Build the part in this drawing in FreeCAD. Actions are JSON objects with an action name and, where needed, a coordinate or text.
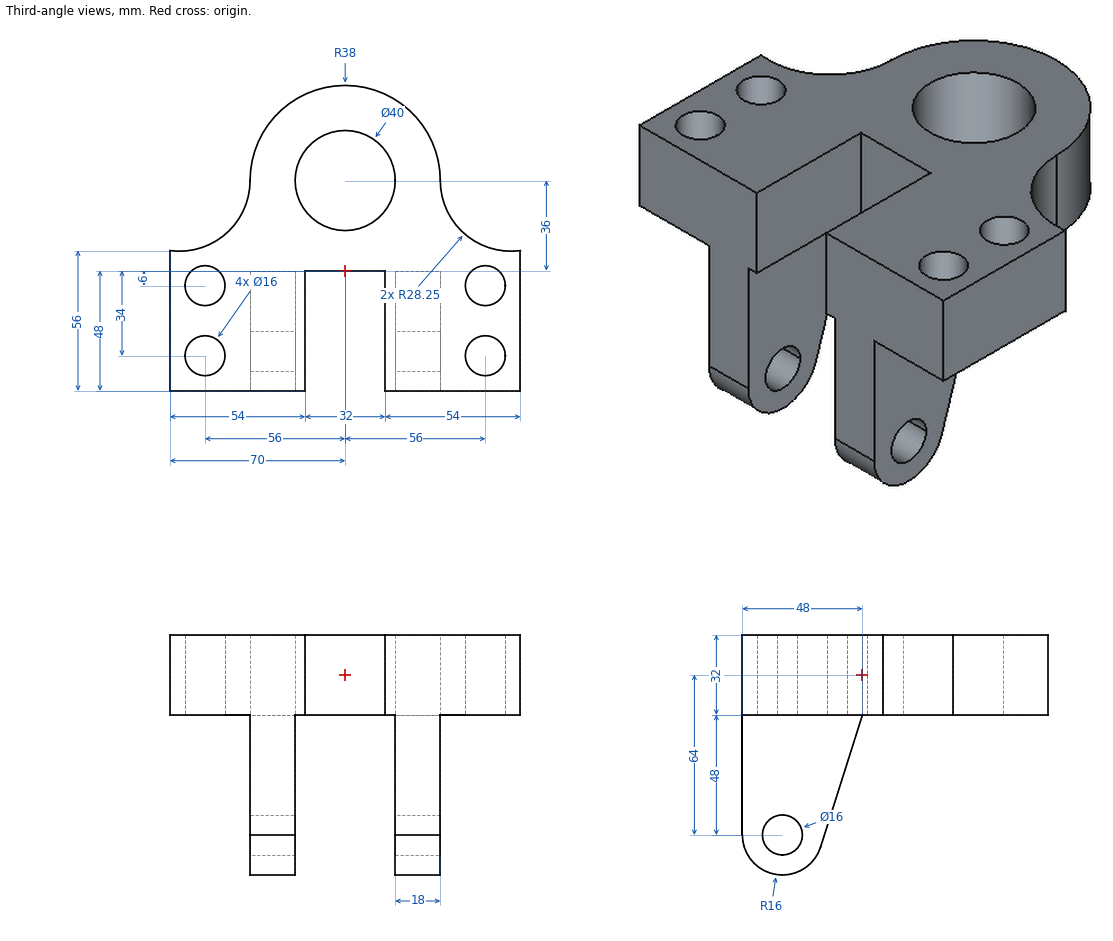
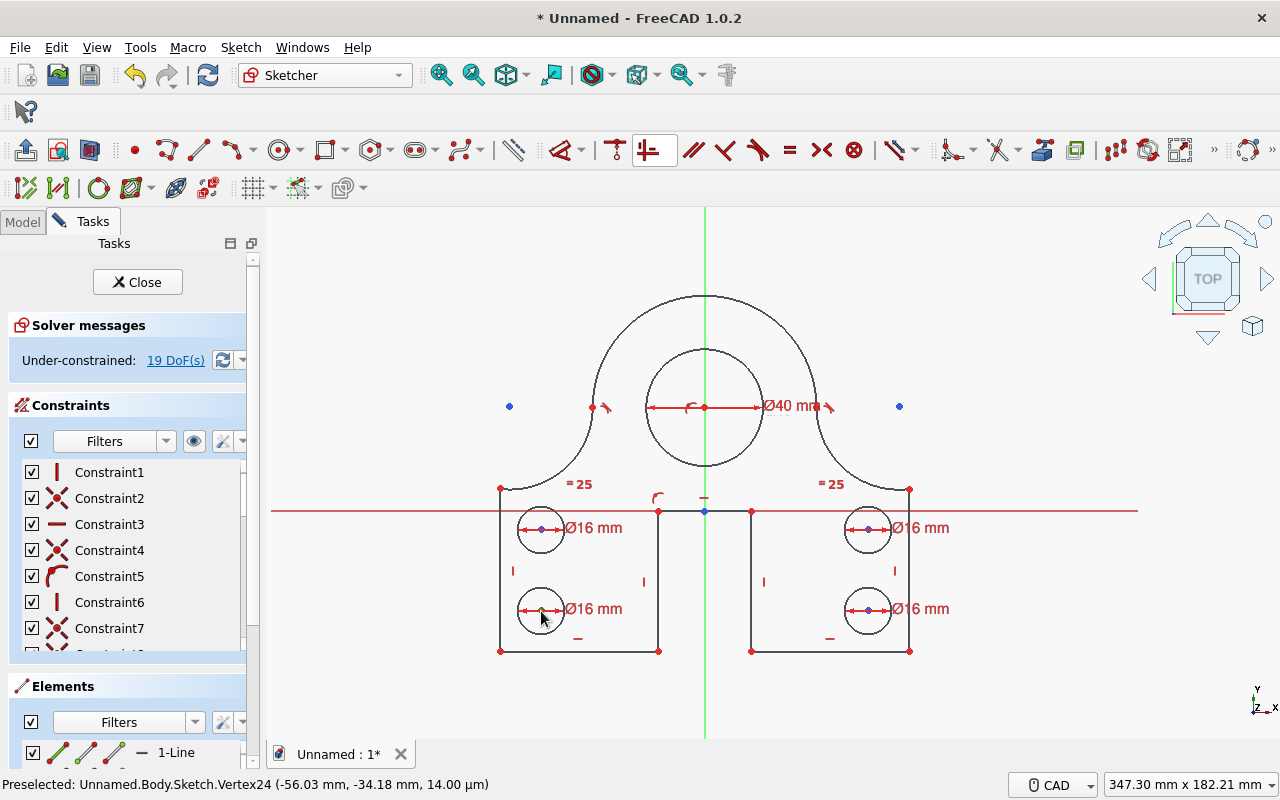
{"action": "left_click", "coordinate": [541, 530]}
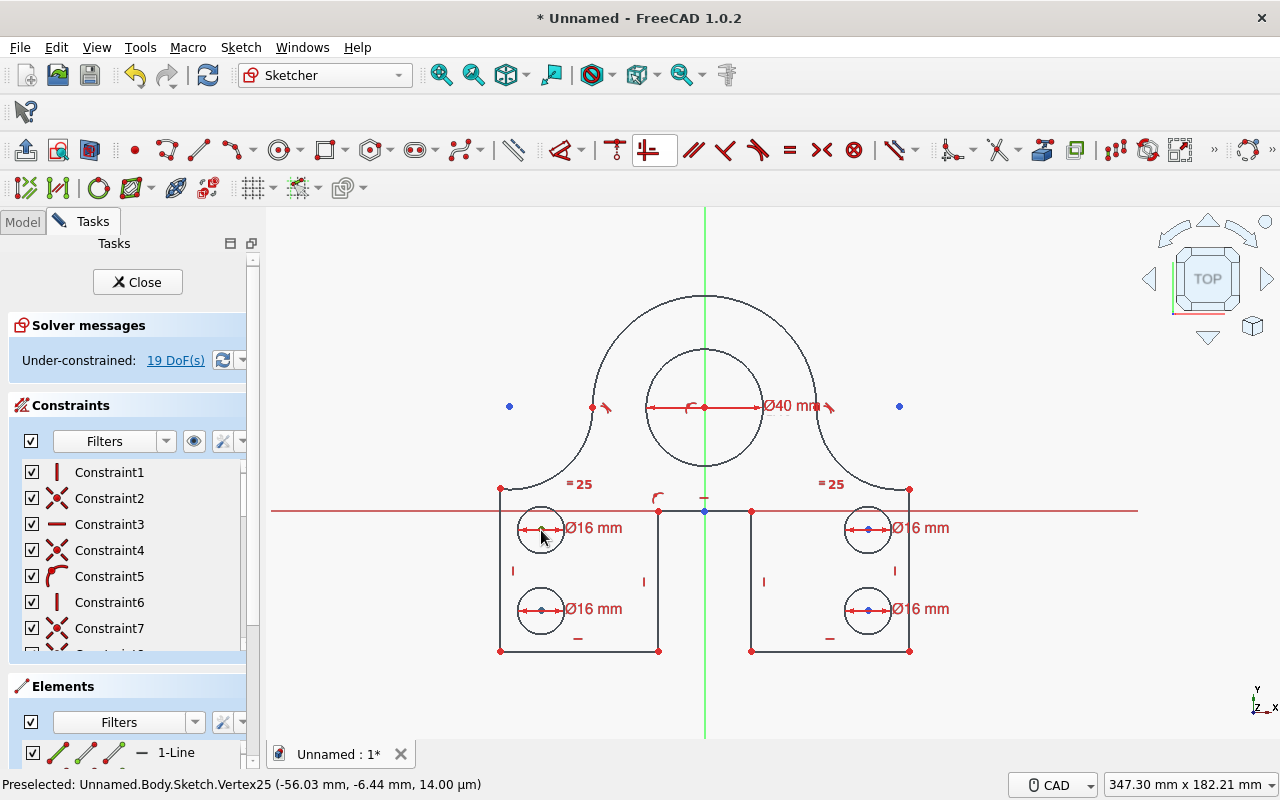
{"action": "key", "text": "v"}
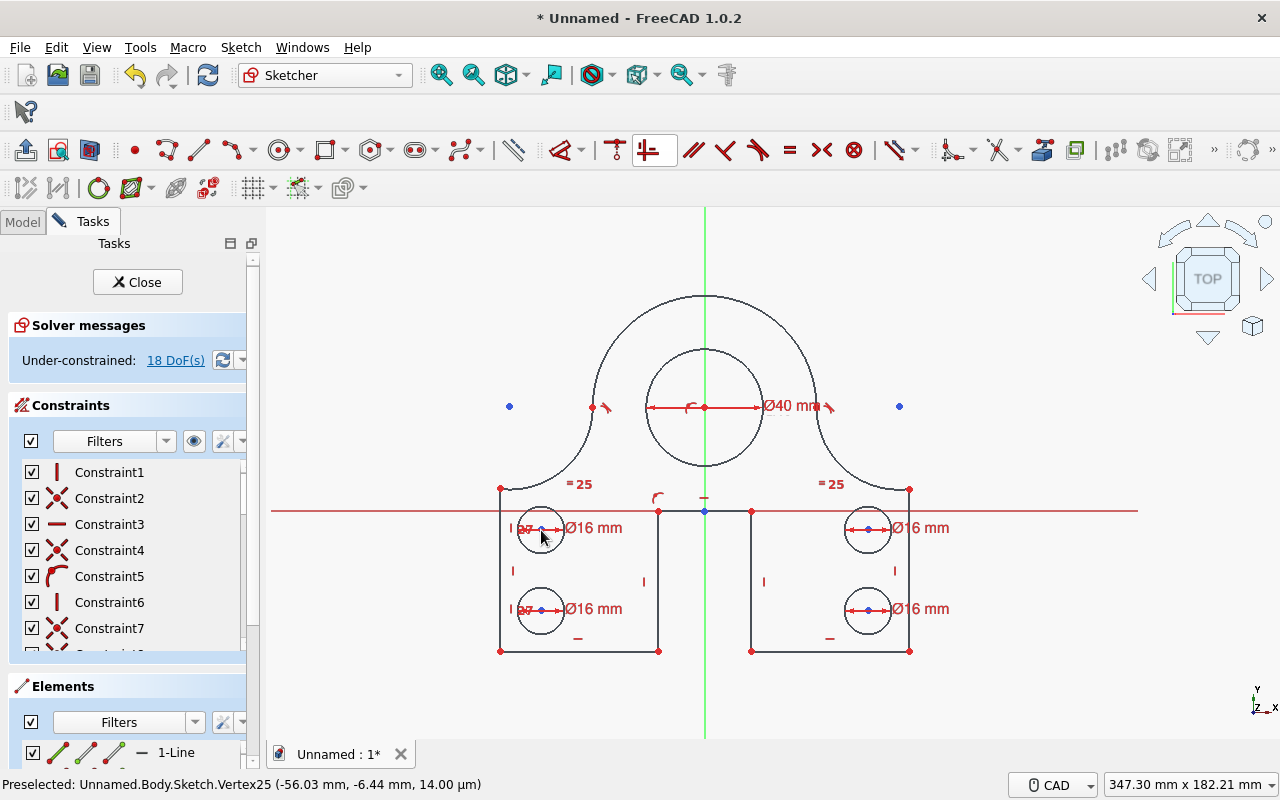
{"action": "left_click", "coordinate": [868, 611]}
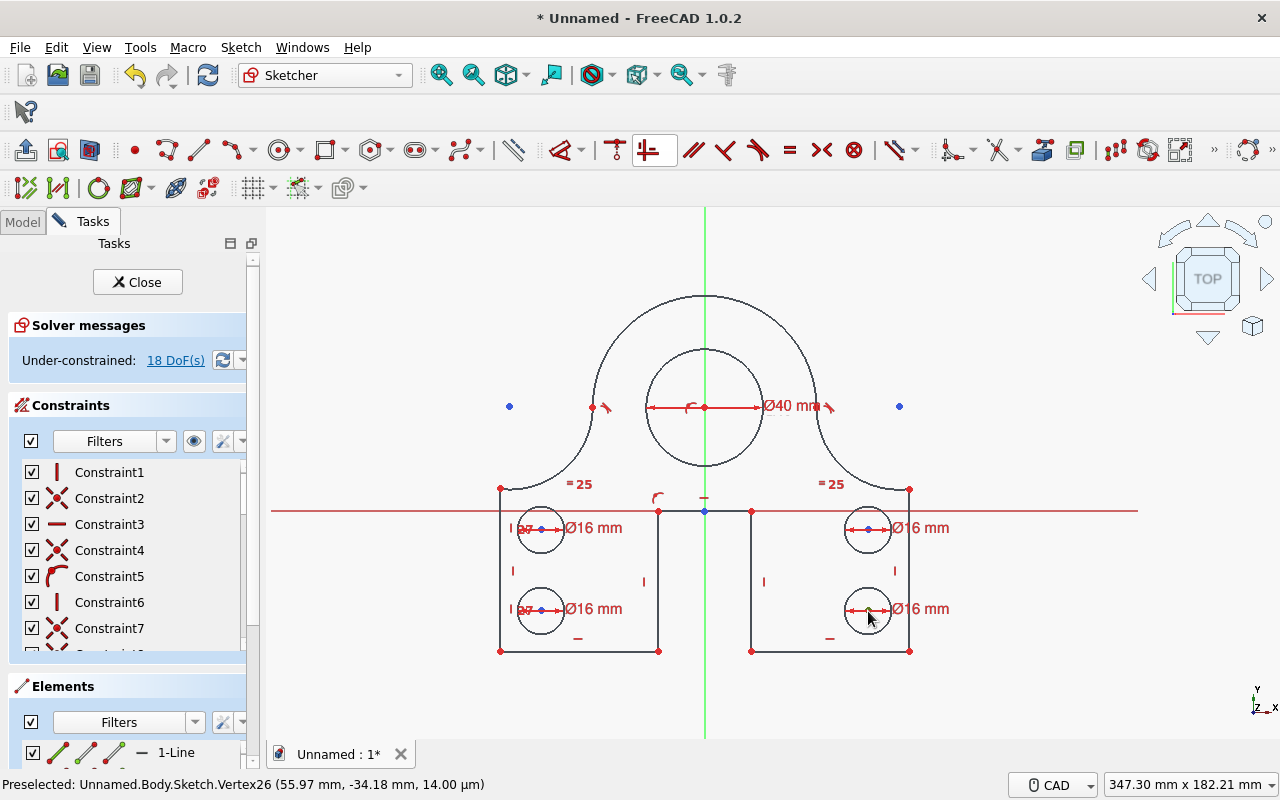
{"action": "left_click", "coordinate": [868, 530]}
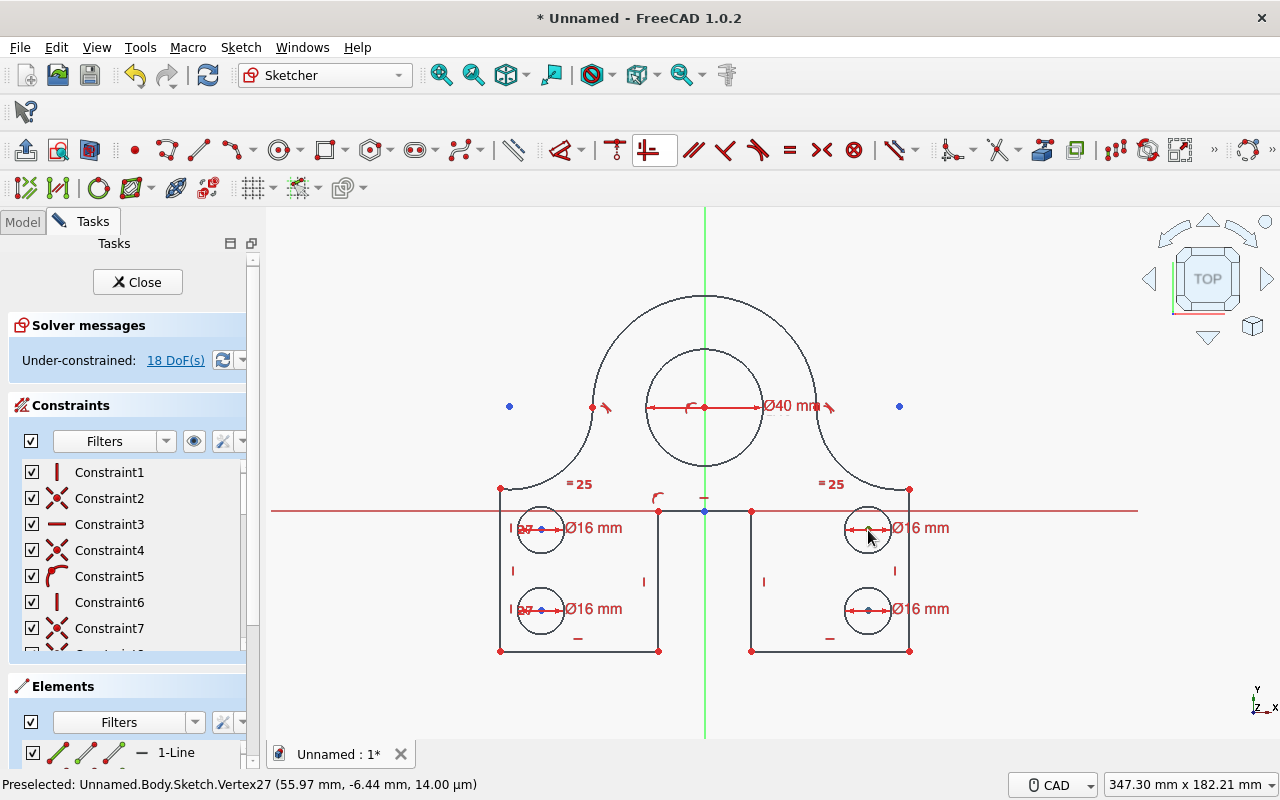
{"action": "left_click", "coordinate": [672, 150]}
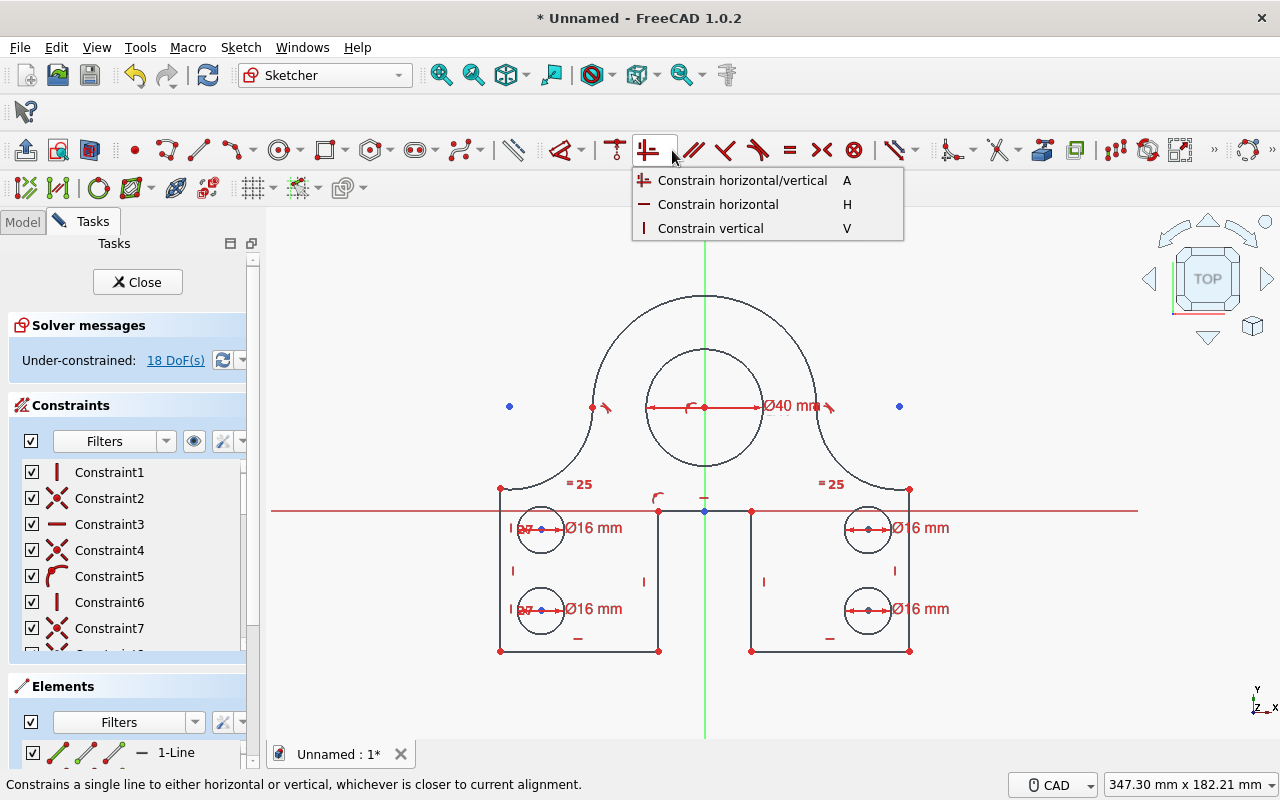
{"action": "left_click", "coordinate": [768, 228]}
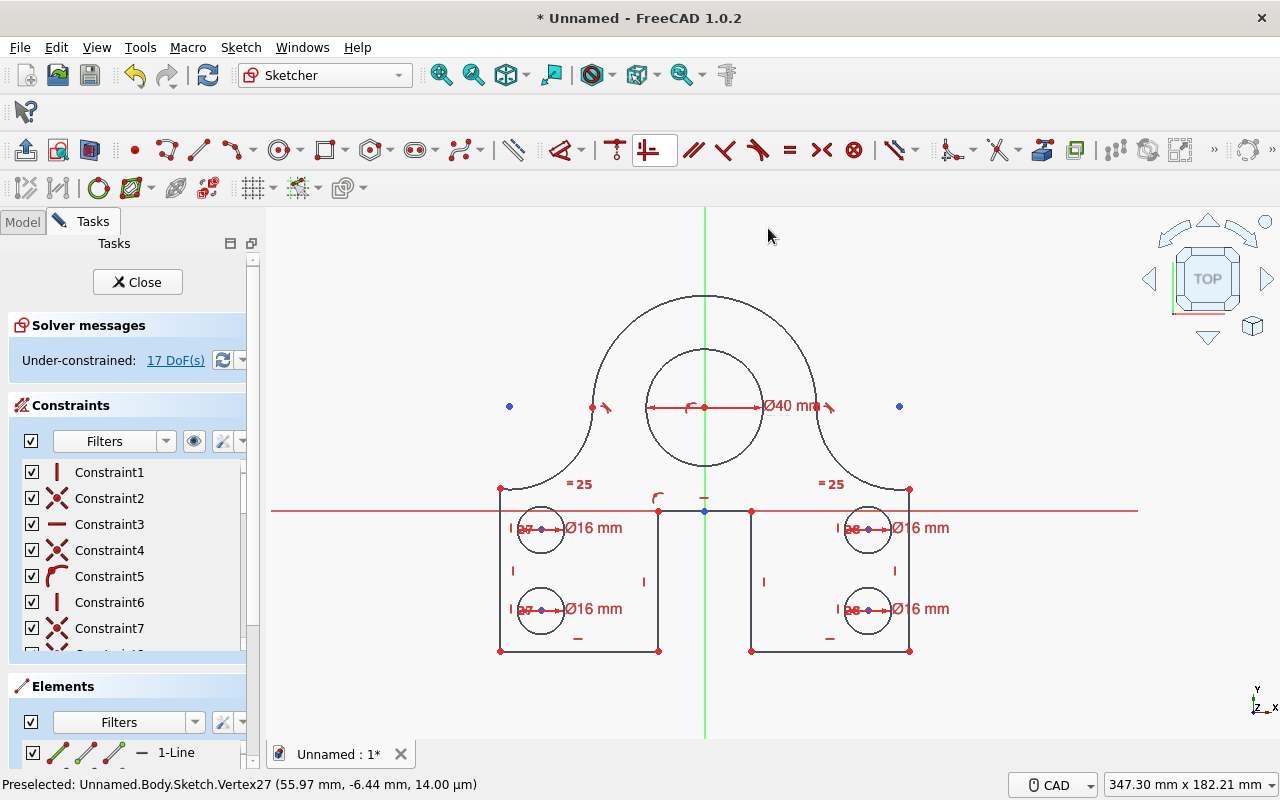
{"action": "left_click", "coordinate": [560, 150]}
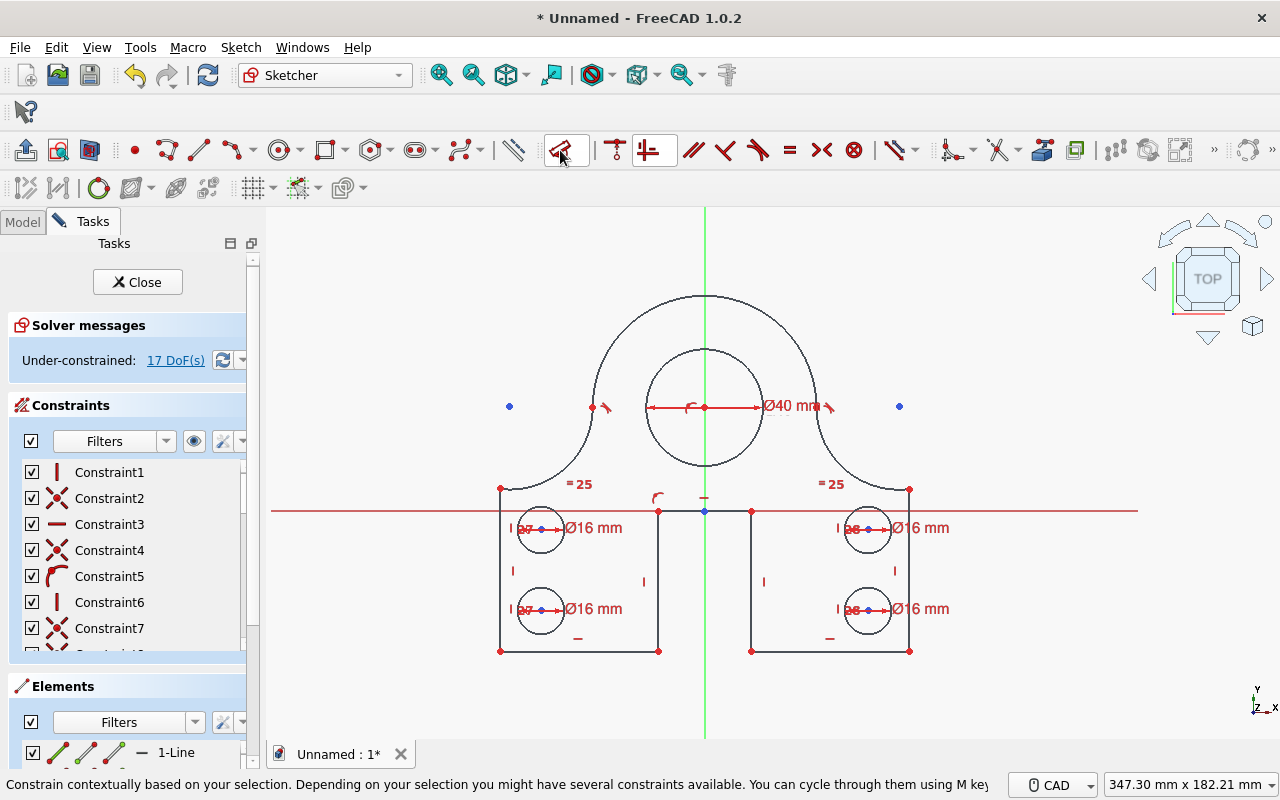
{"action": "left_click", "coordinate": [827, 447]}
{"action": "left_click", "coordinate": [799, 463]}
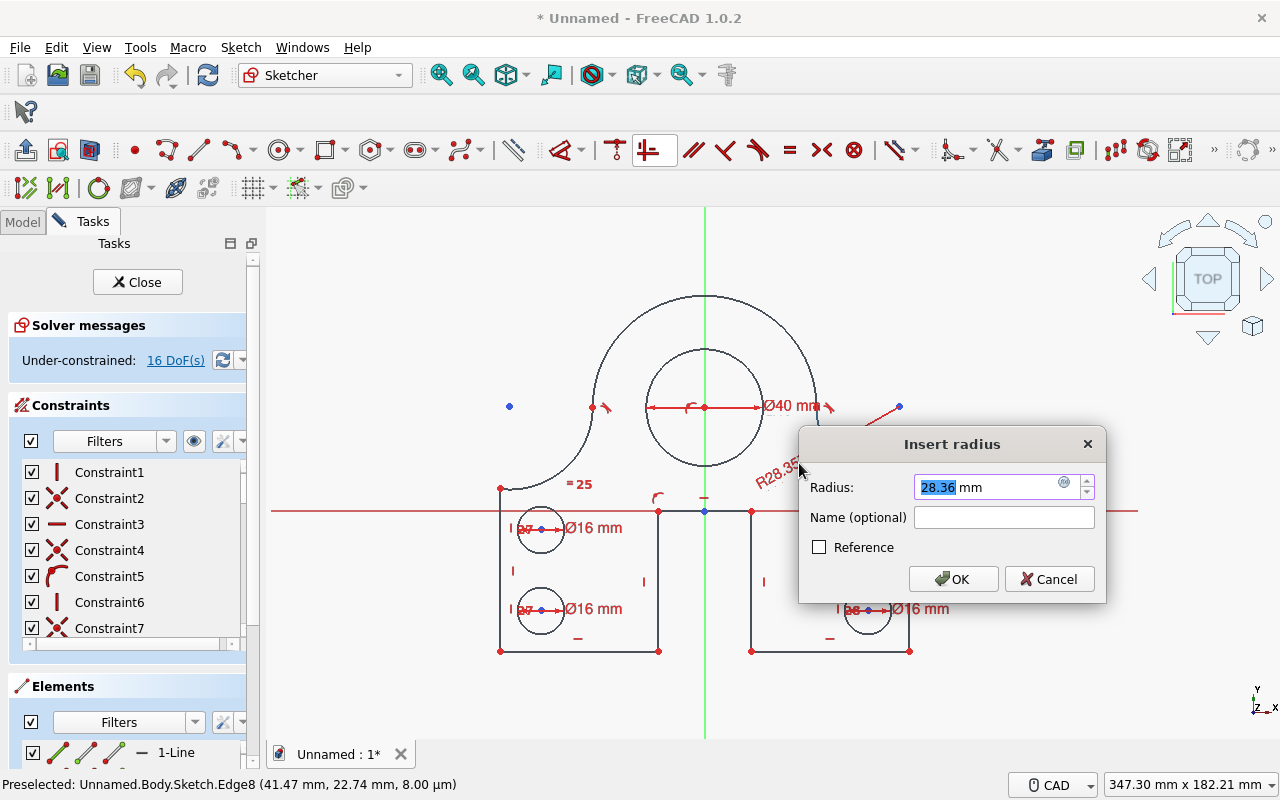
{"action": "type", "text": "28.25"}
{"action": "key", "text": "Return"}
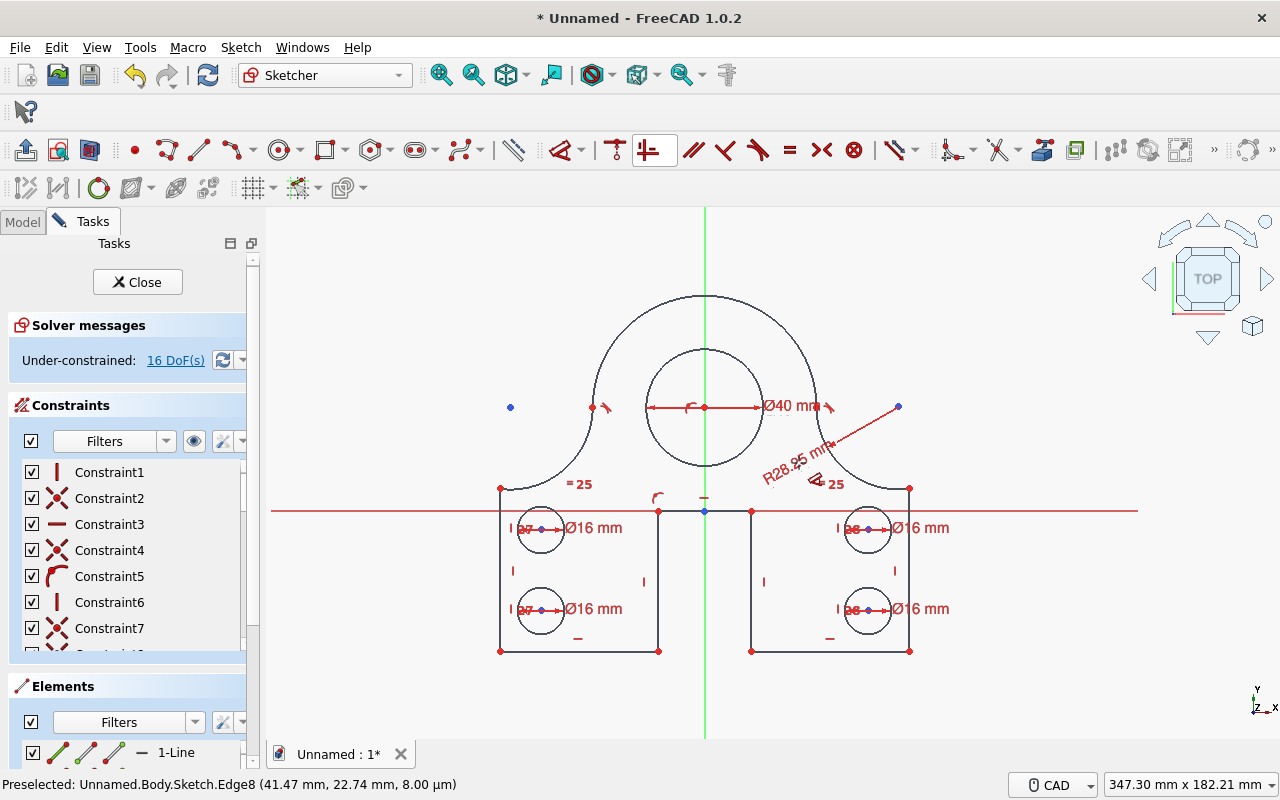
{"action": "left_click", "coordinate": [770, 317]}
{"action": "left_click", "coordinate": [789, 291]}